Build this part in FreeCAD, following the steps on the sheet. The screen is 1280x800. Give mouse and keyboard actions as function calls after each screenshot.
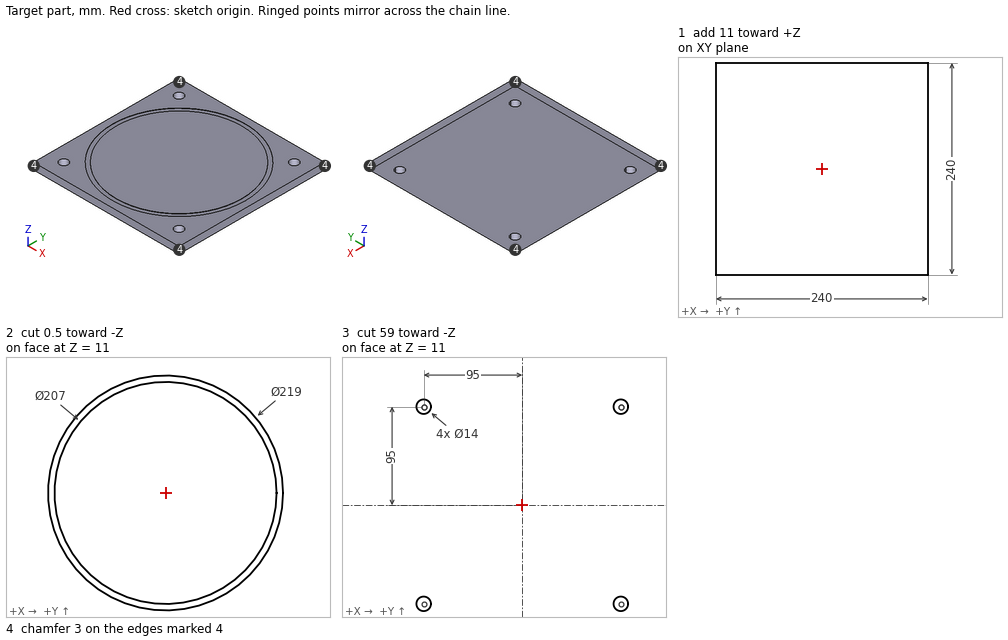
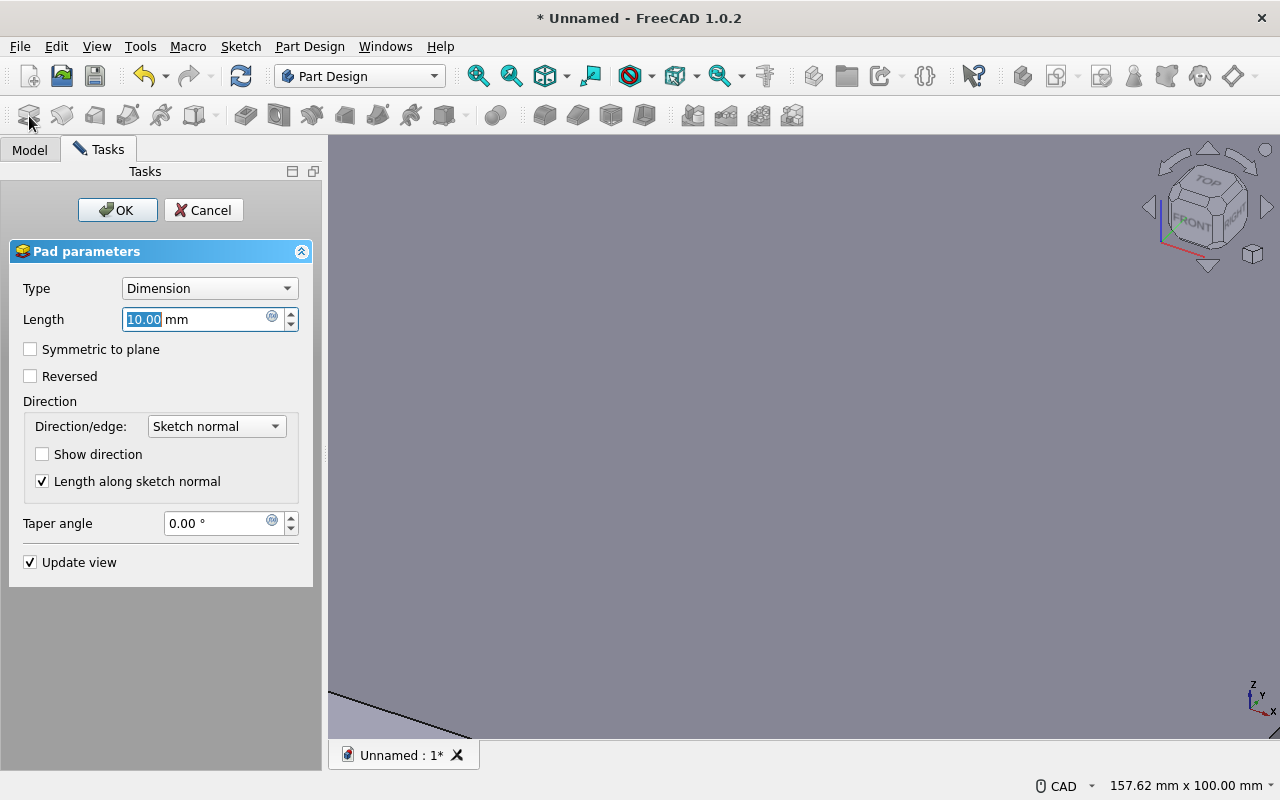
text(11)
key(Tab)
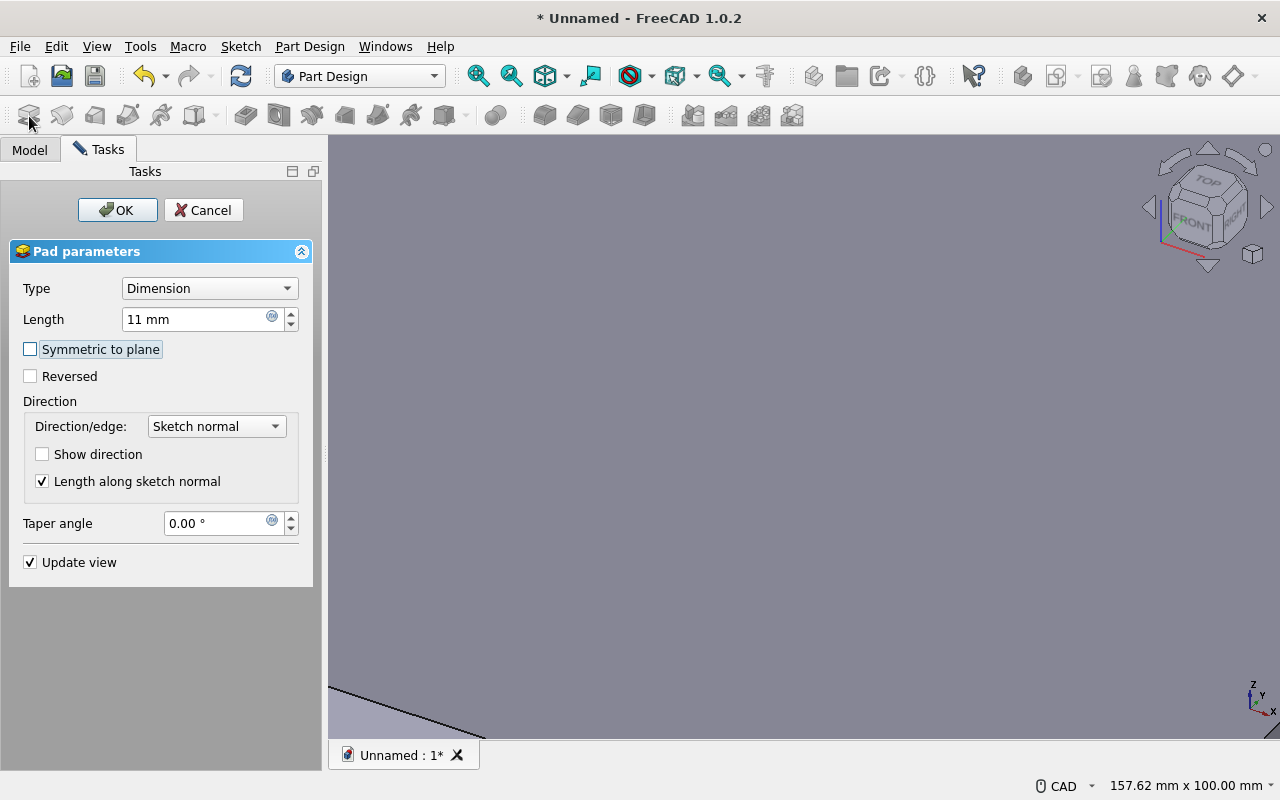
click(118, 210)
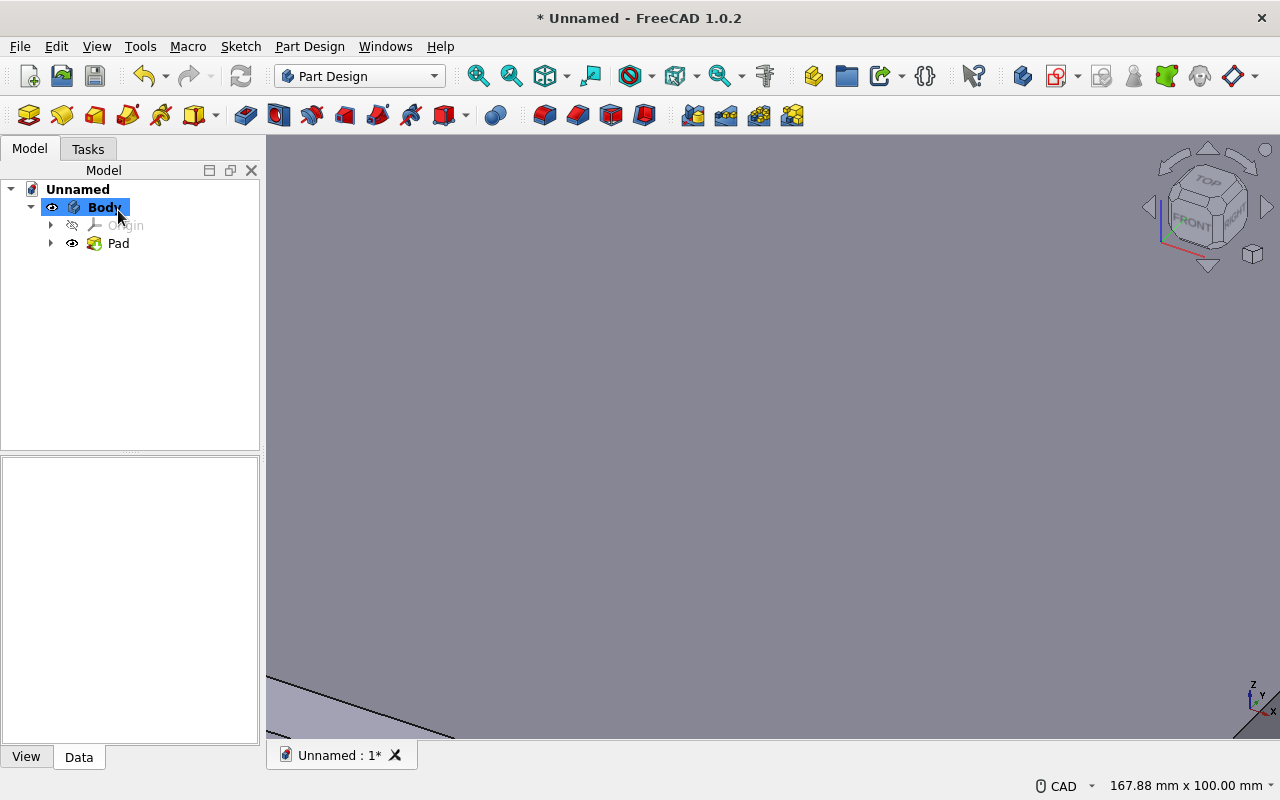
click(479, 76)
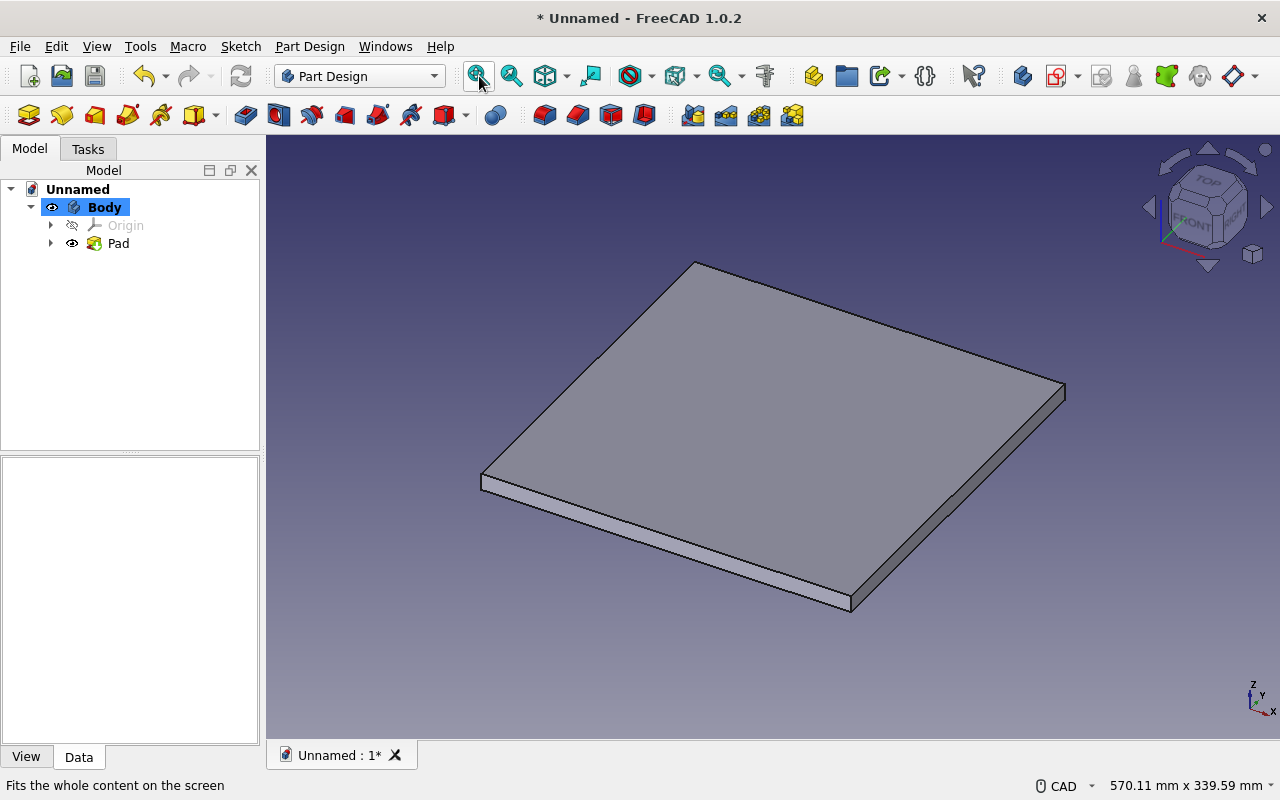
click(773, 428)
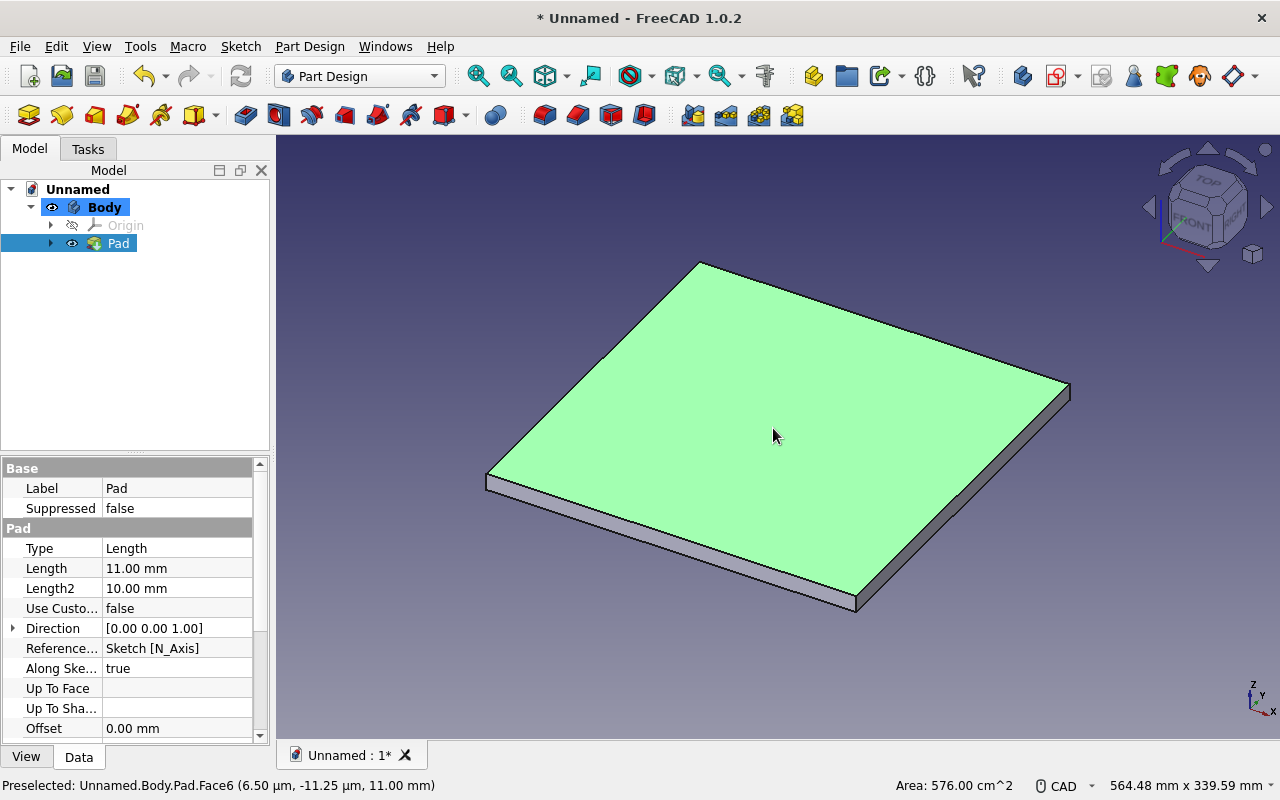
click(1056, 76)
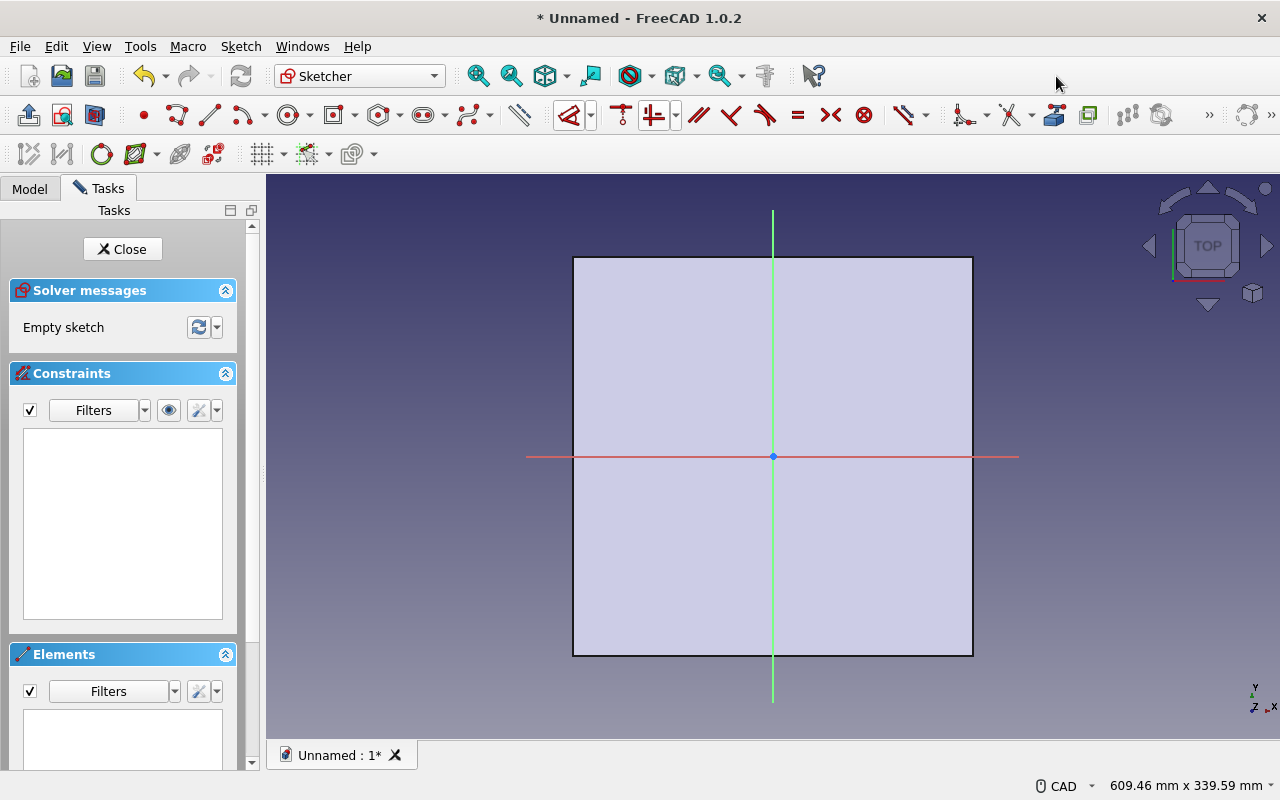
click(288, 116)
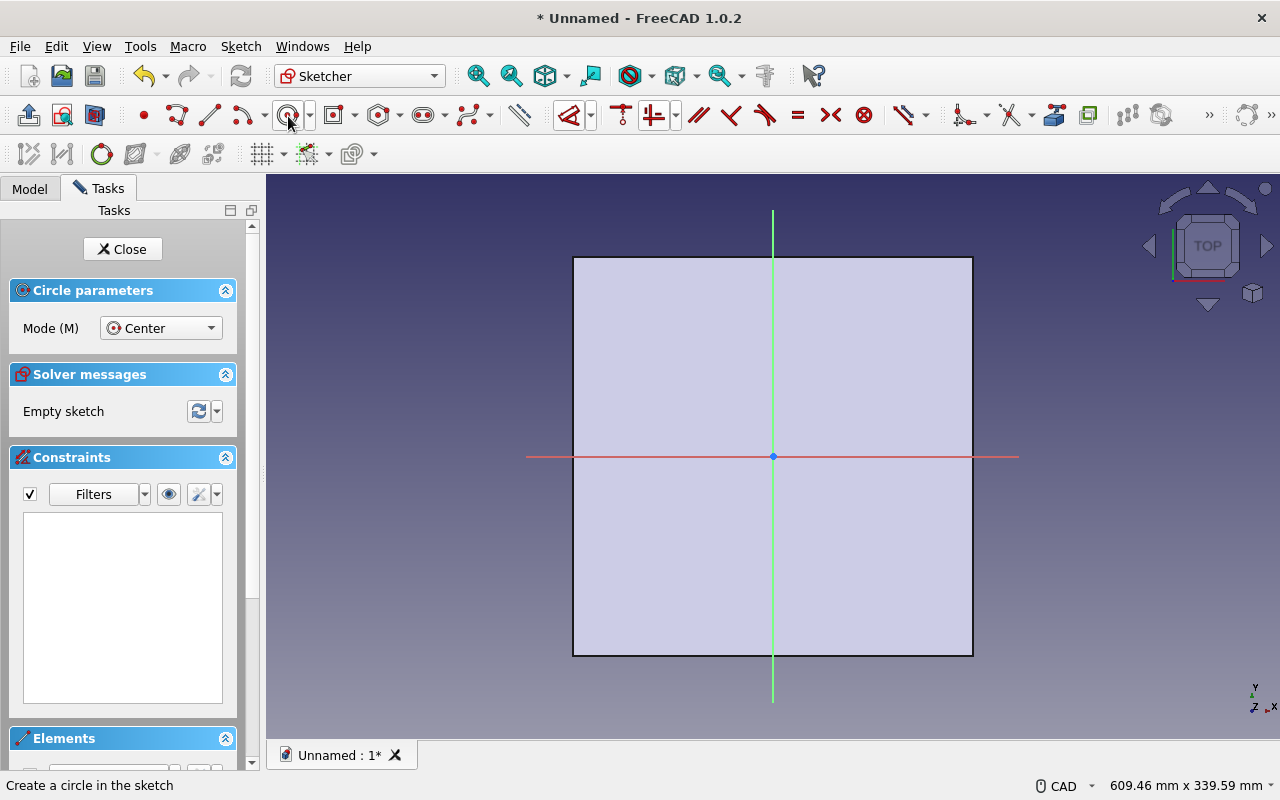
click(773, 456)
move(902, 328)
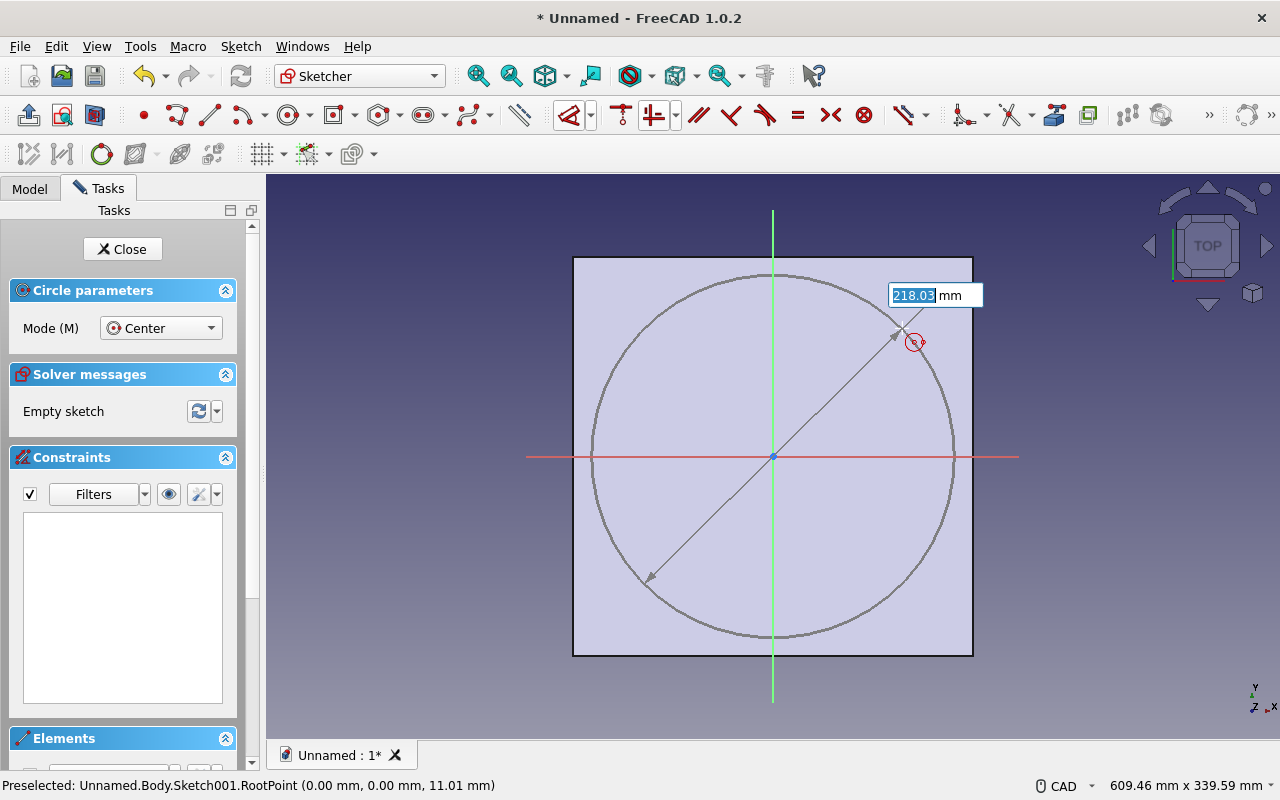
text(219)
key(Return)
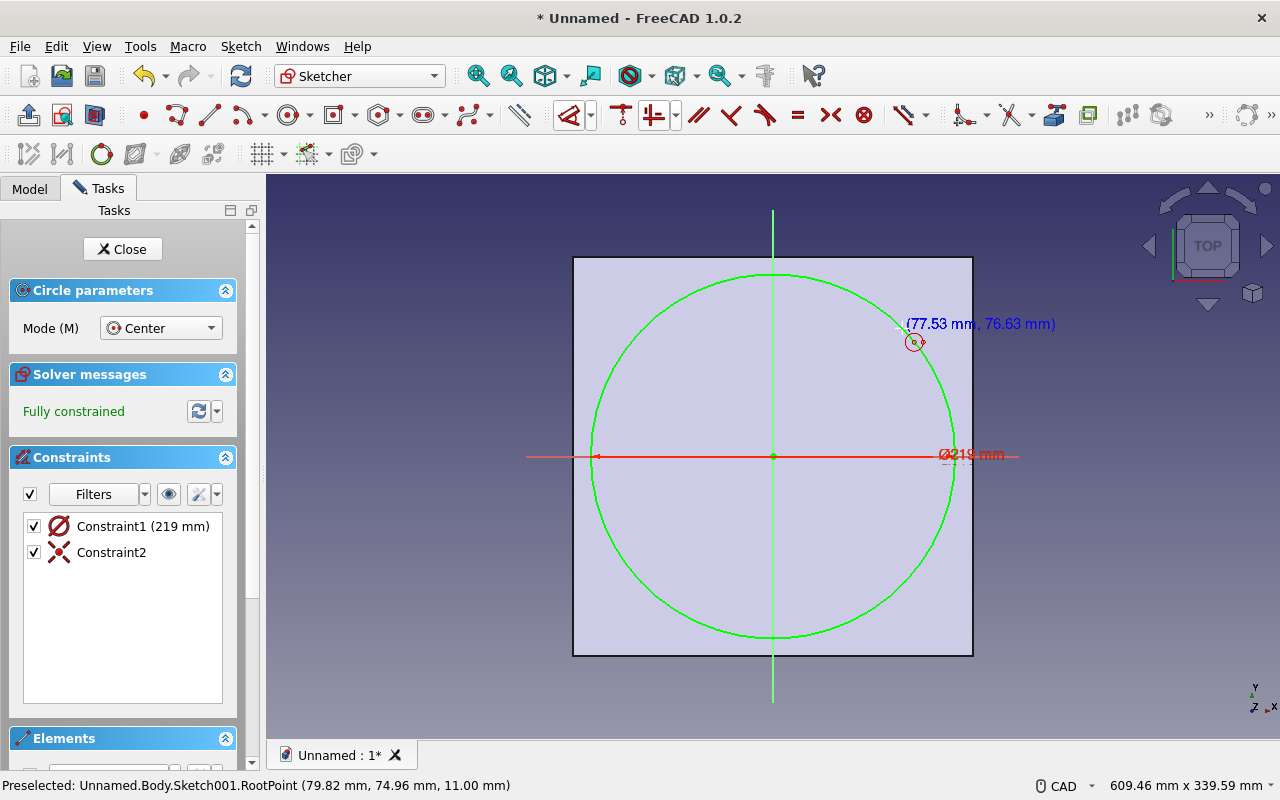
click(773, 456)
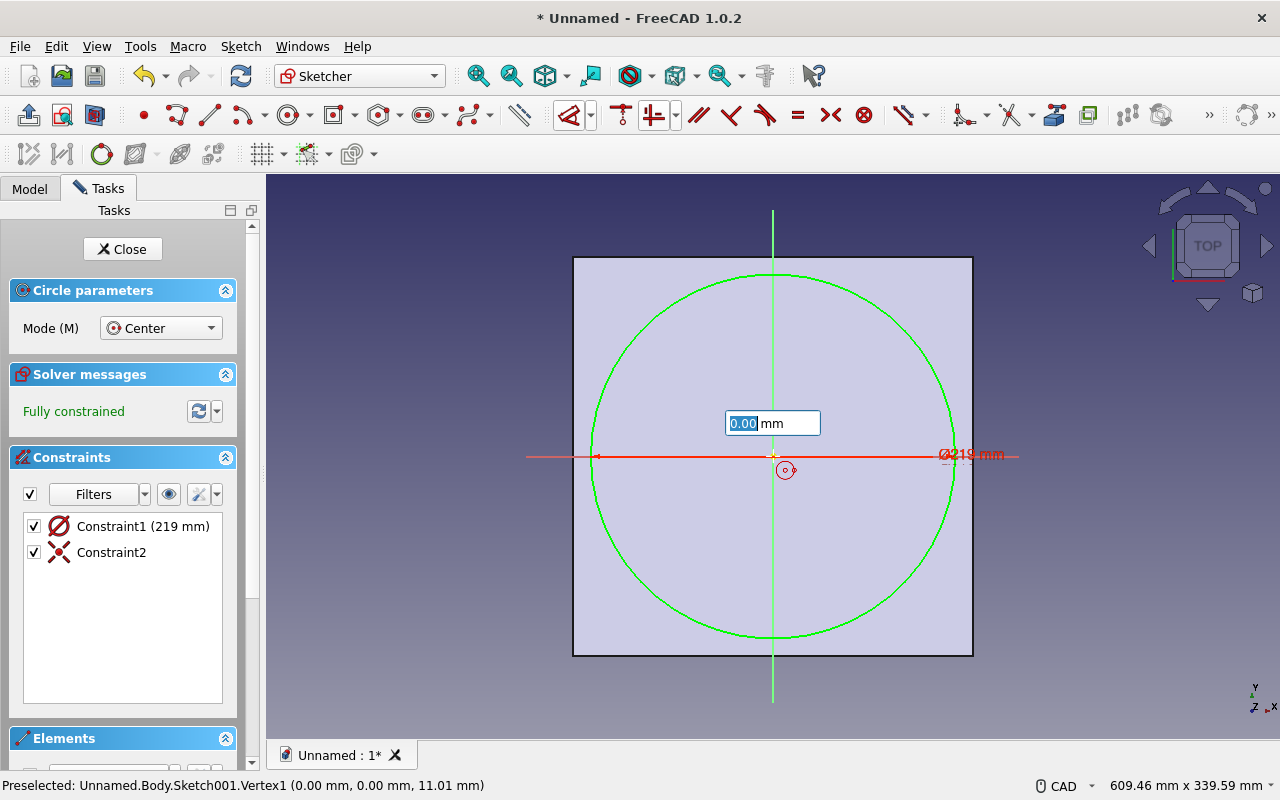
scroll(895, 335, up, 3)
move(894, 334)